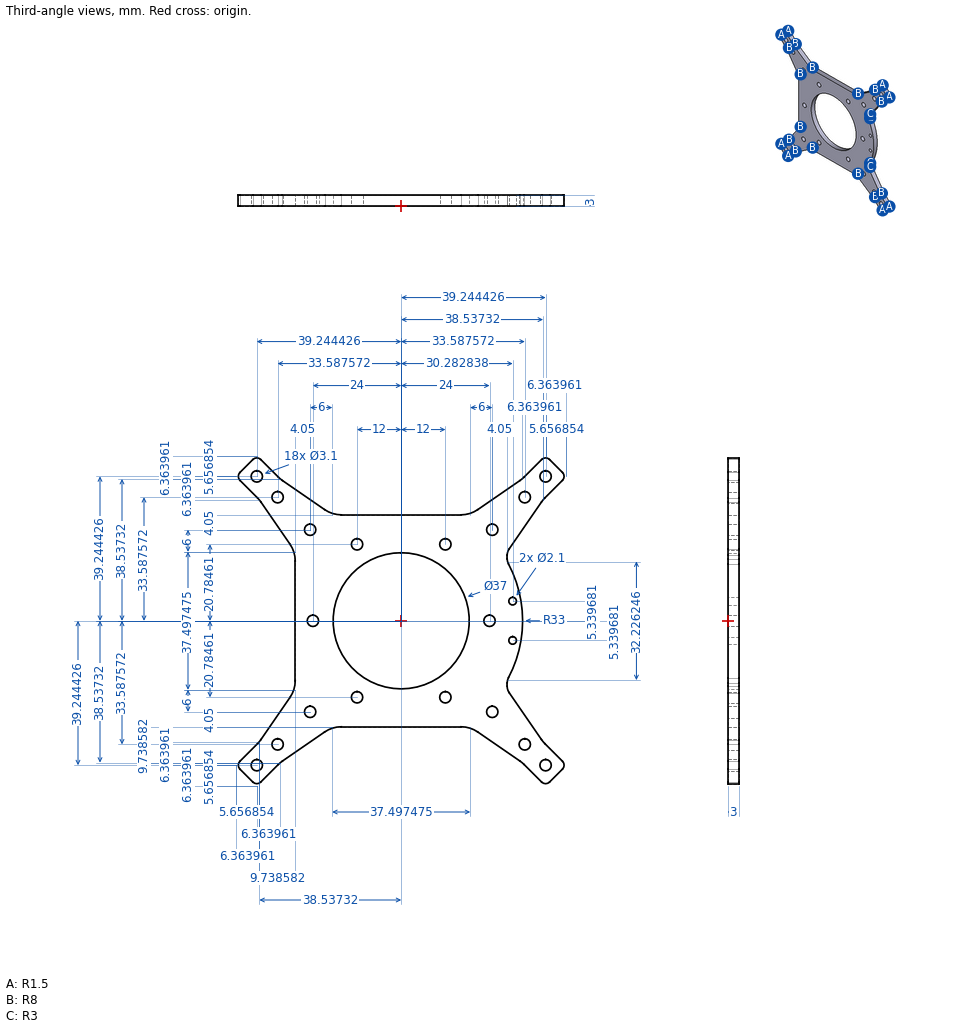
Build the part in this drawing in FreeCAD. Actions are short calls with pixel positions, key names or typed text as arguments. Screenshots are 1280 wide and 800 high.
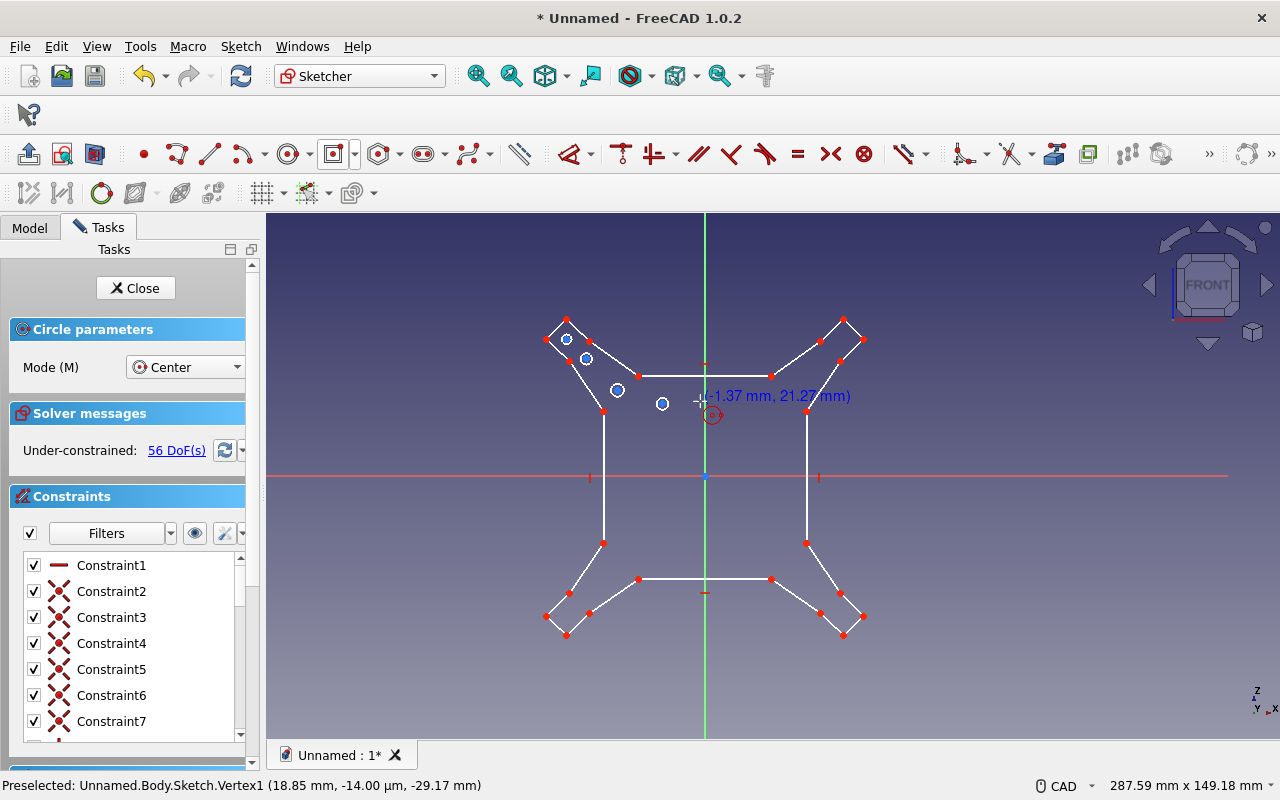
click(748, 403)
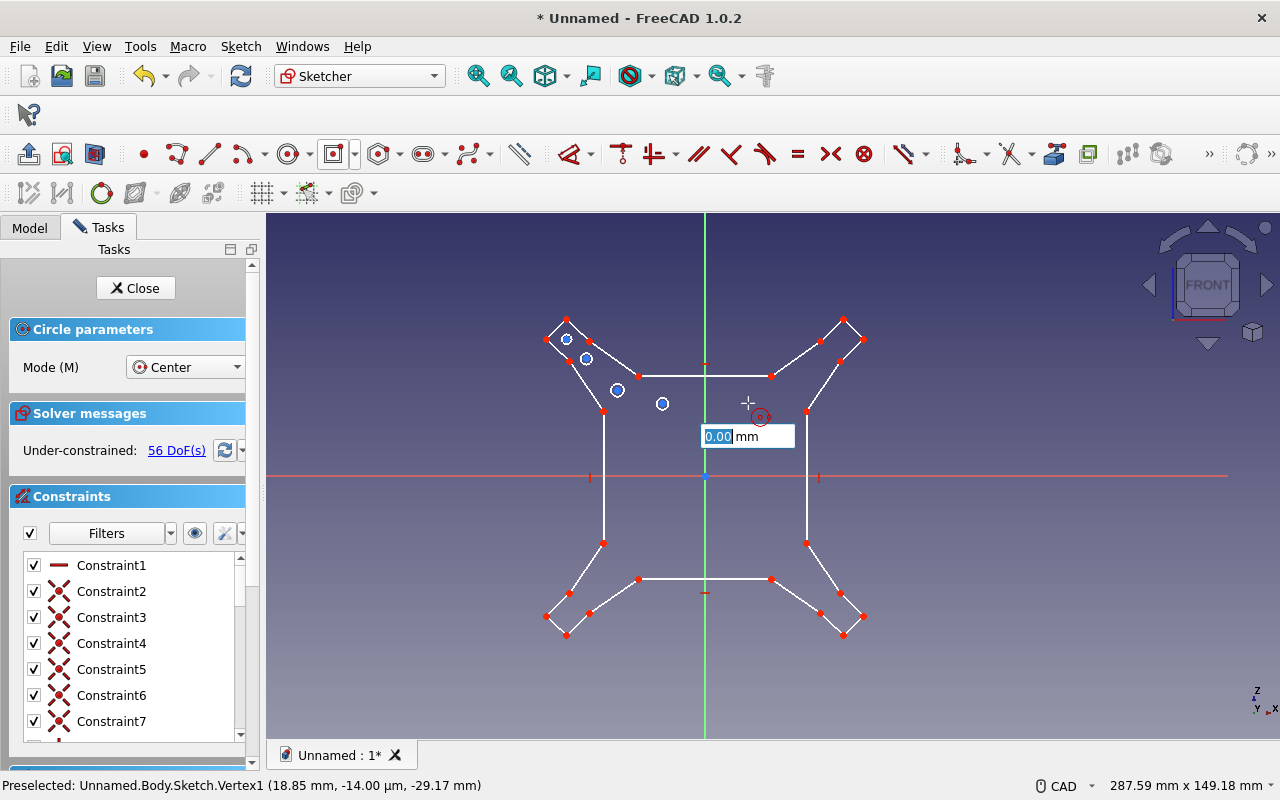
scroll(751, 399, up, 6)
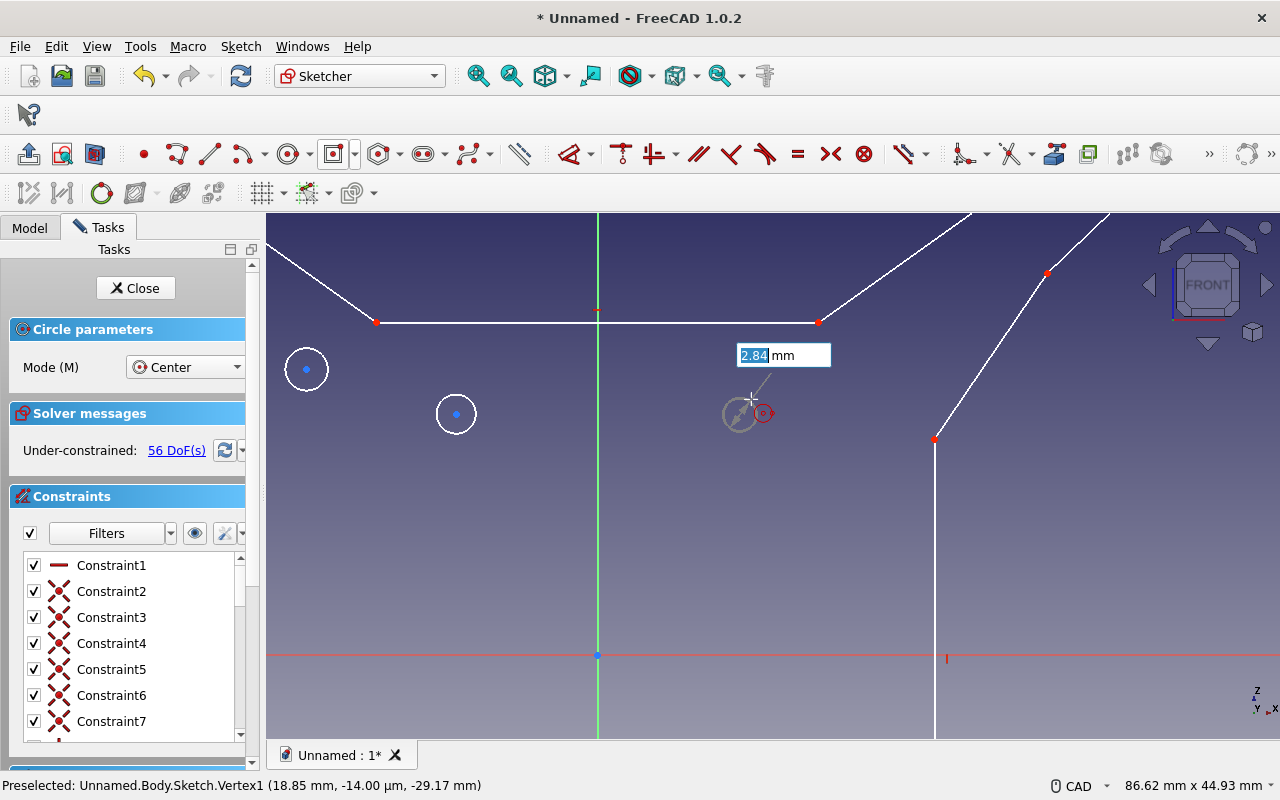
click(751, 399)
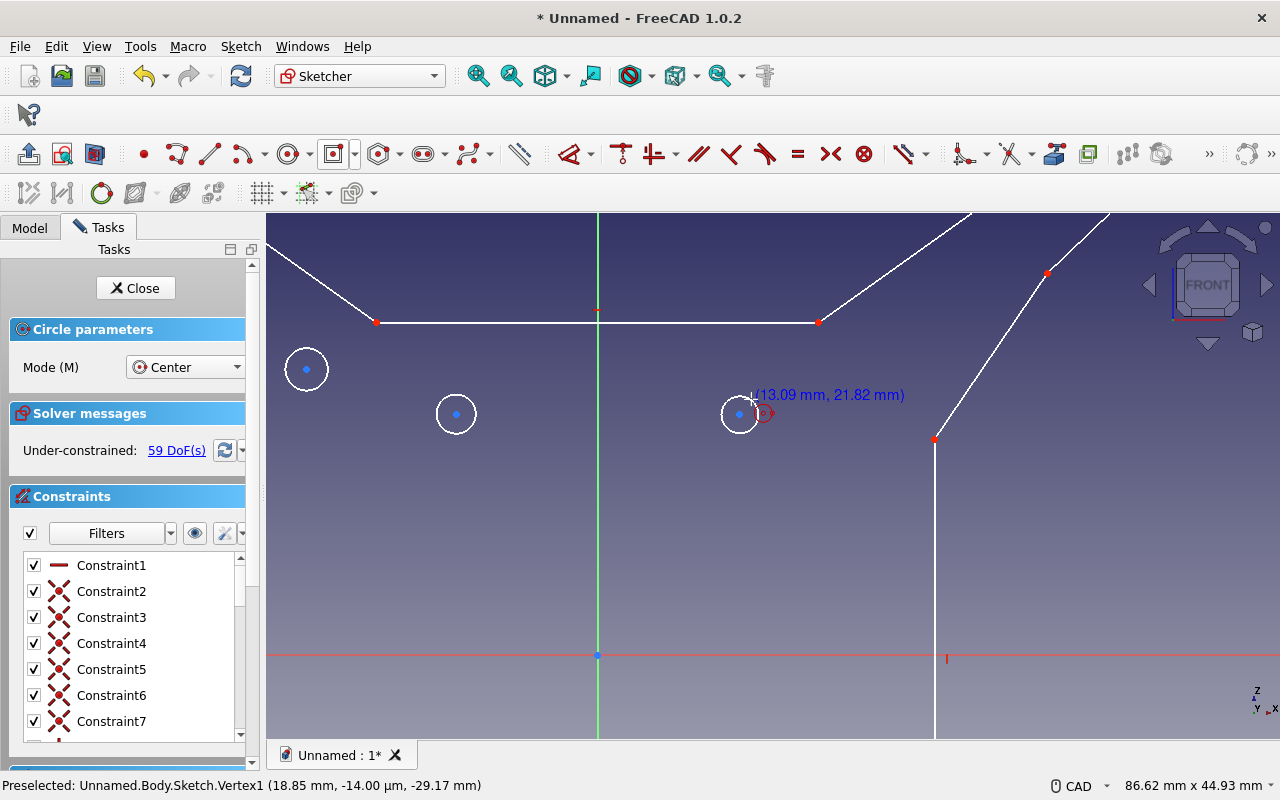
scroll(750, 399, down, 6)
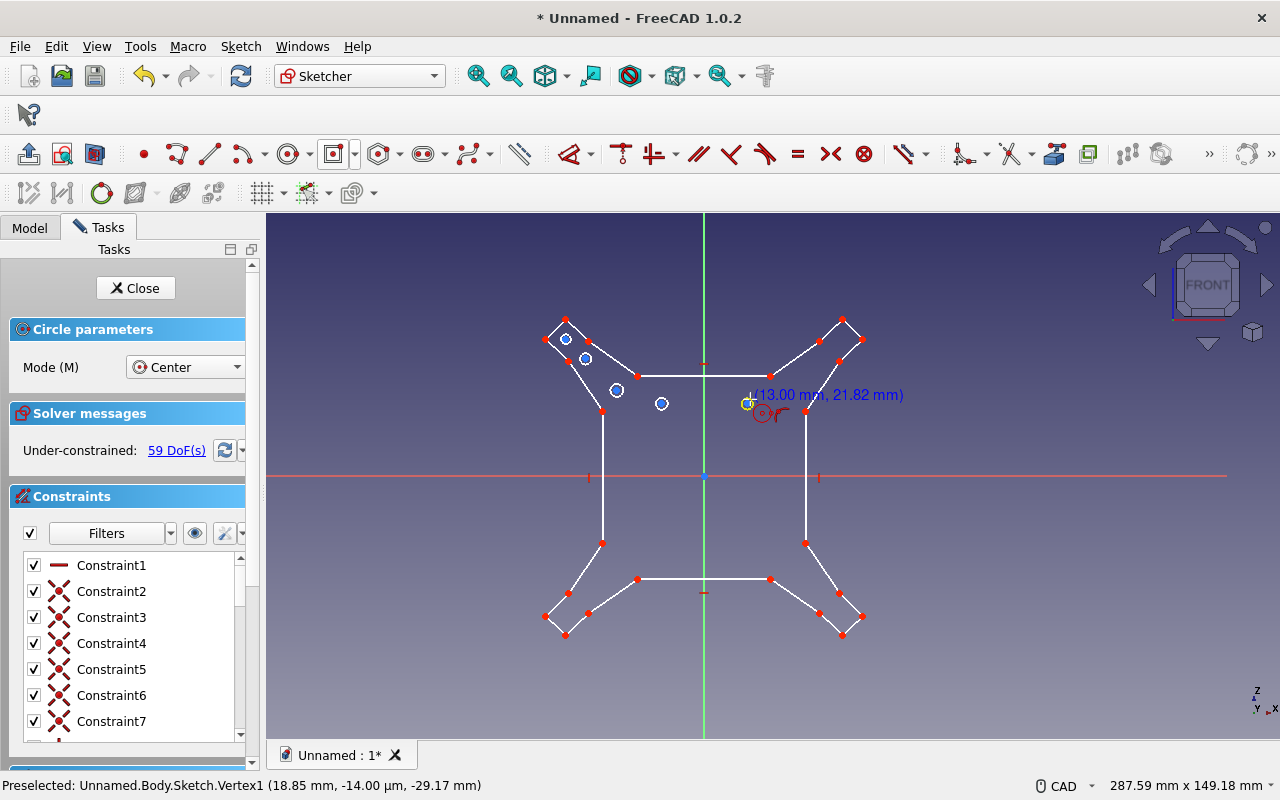
scroll(843, 338, up, 8)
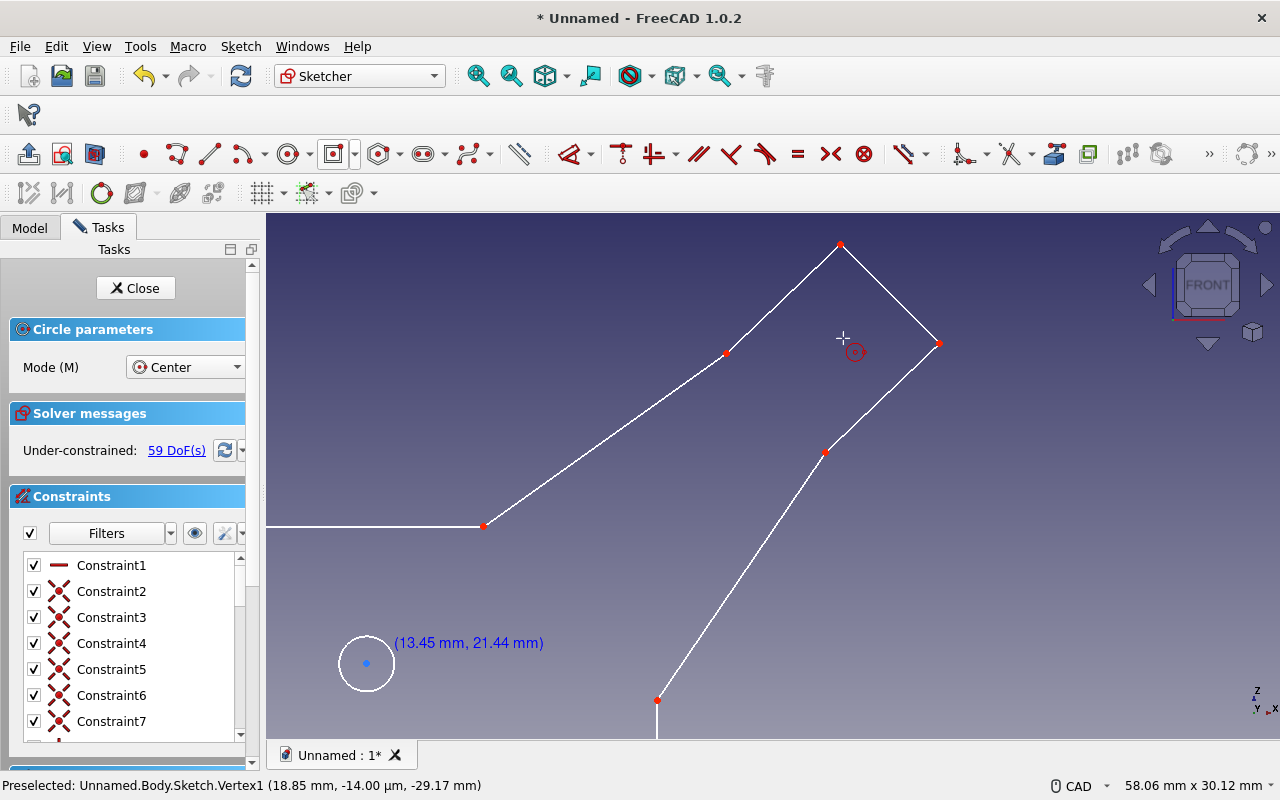
scroll(844, 338, down, 8)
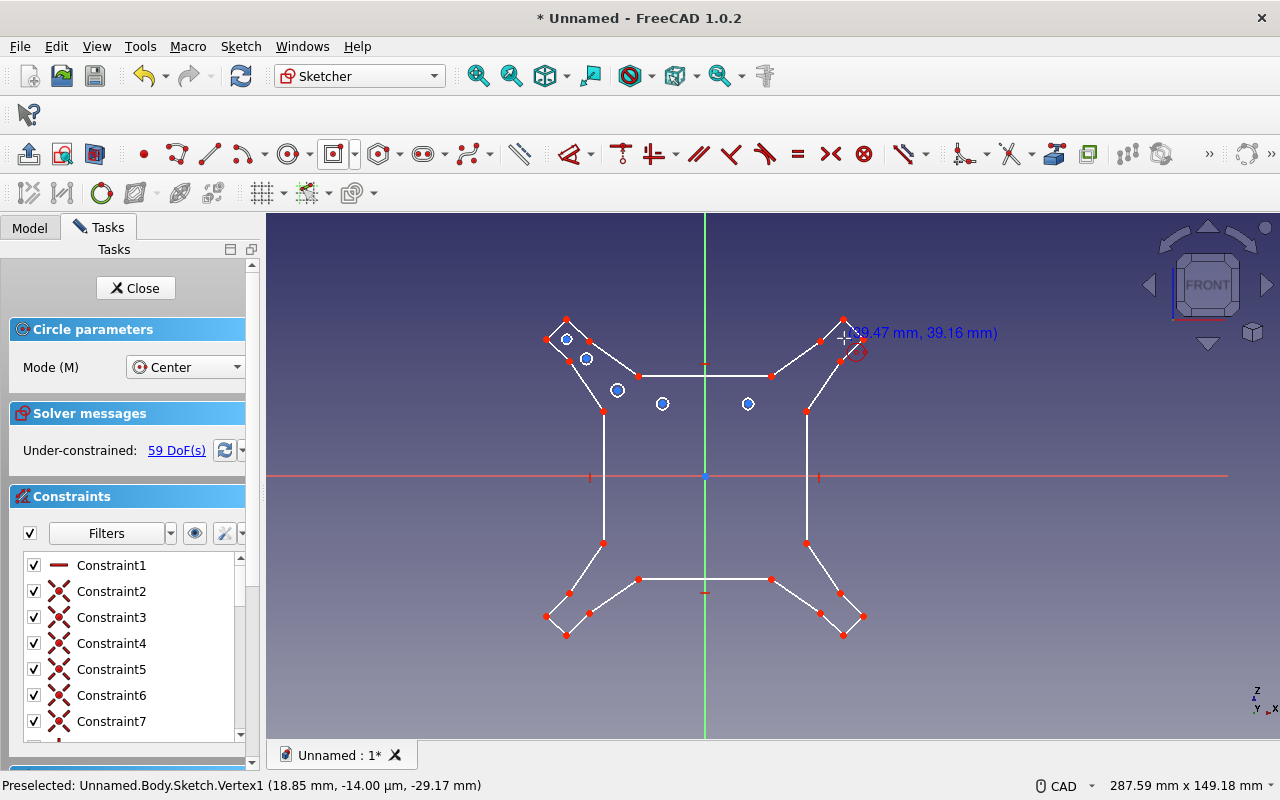
click(844, 338)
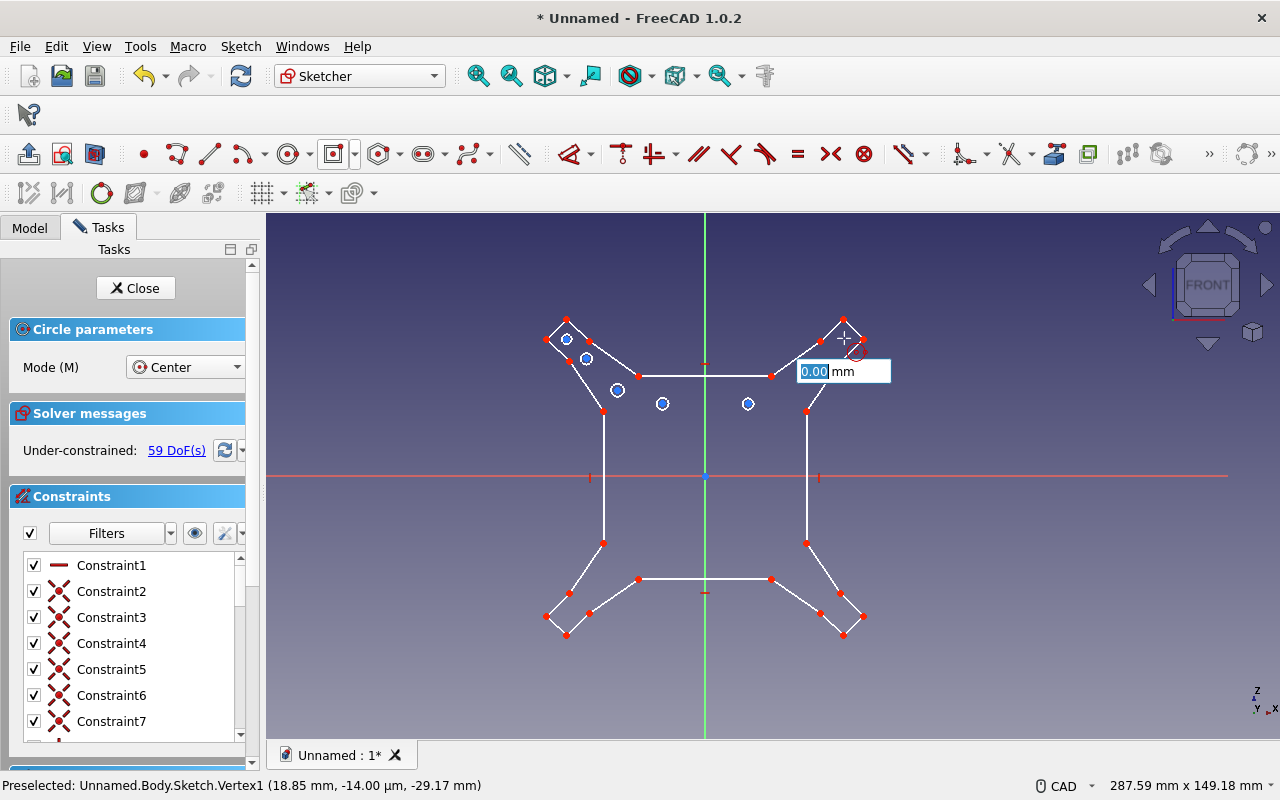
scroll(840, 342, up, 6)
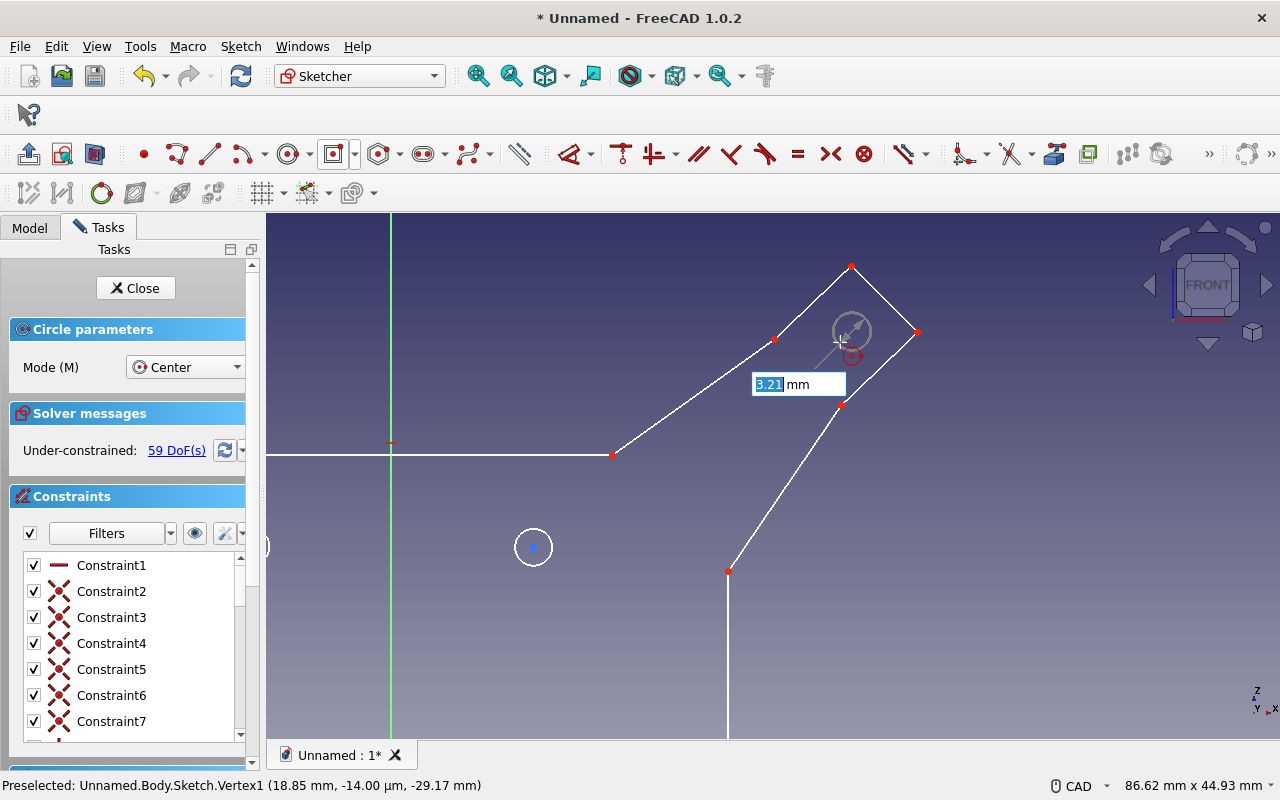
click(838, 341)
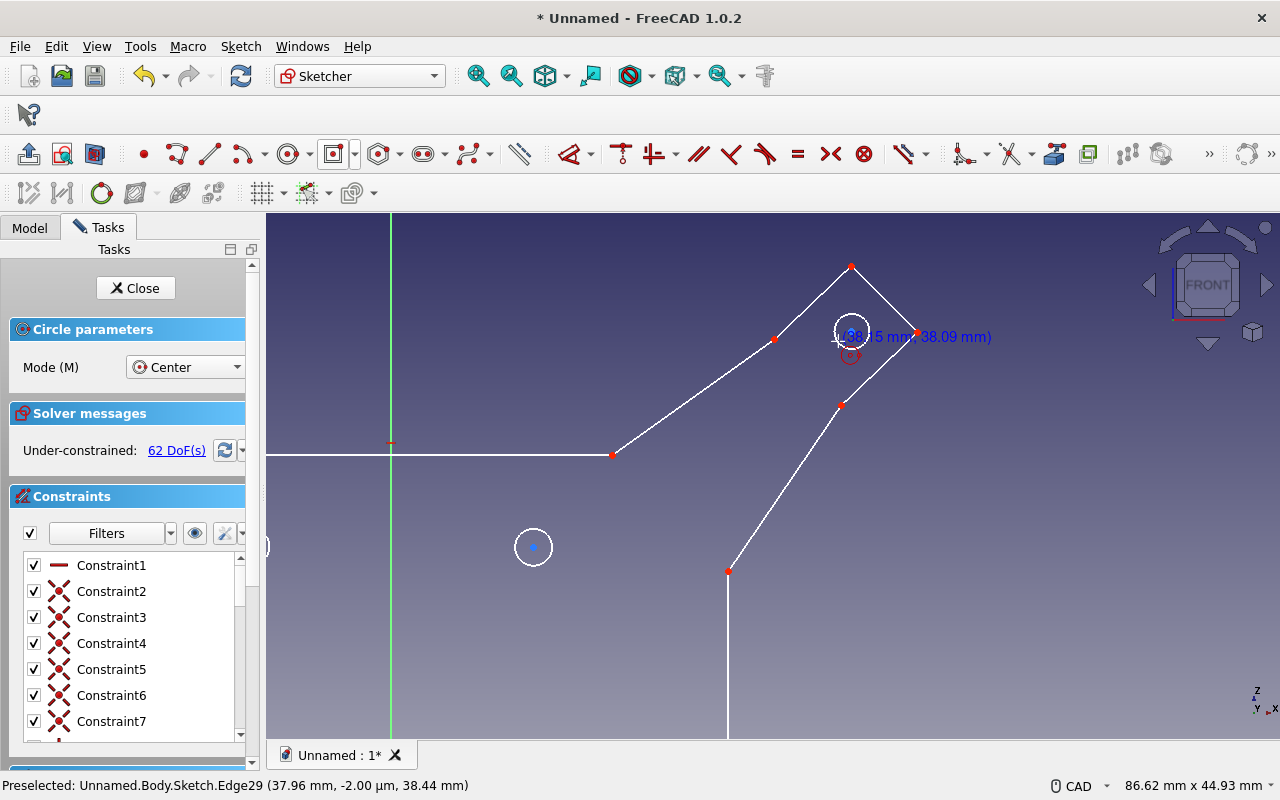
scroll(785, 395, up, 2)